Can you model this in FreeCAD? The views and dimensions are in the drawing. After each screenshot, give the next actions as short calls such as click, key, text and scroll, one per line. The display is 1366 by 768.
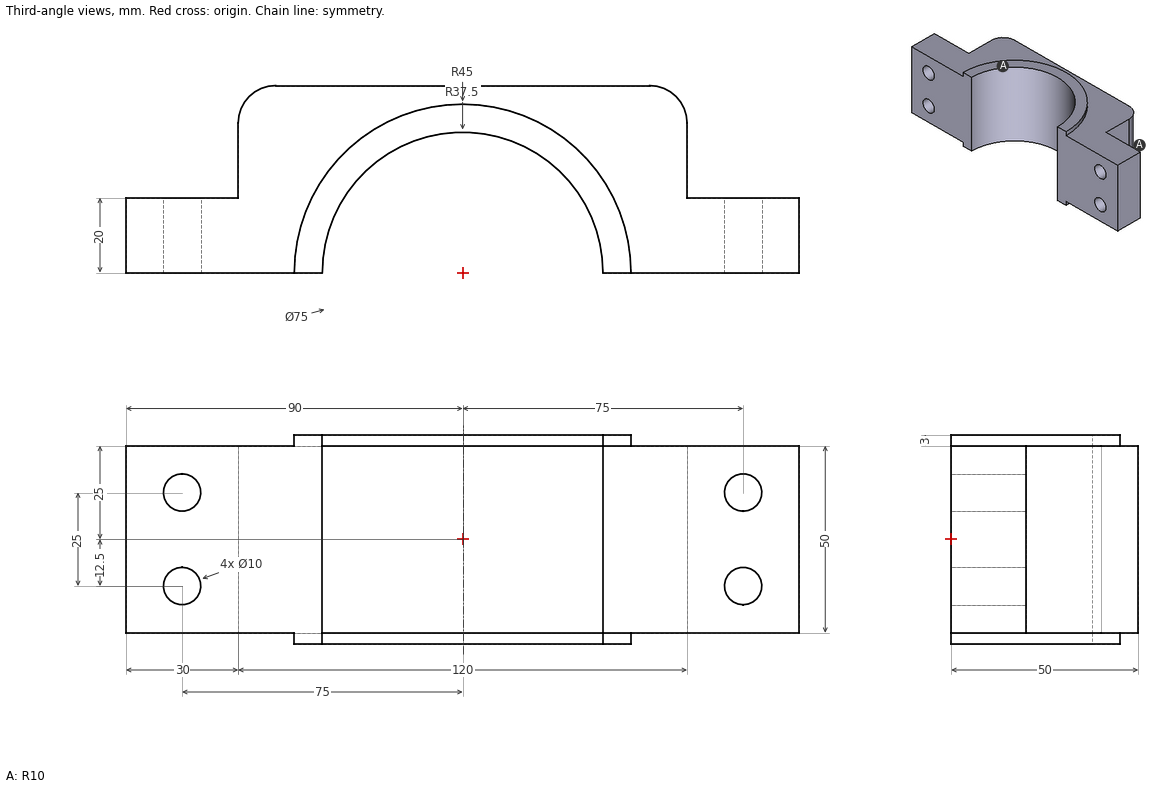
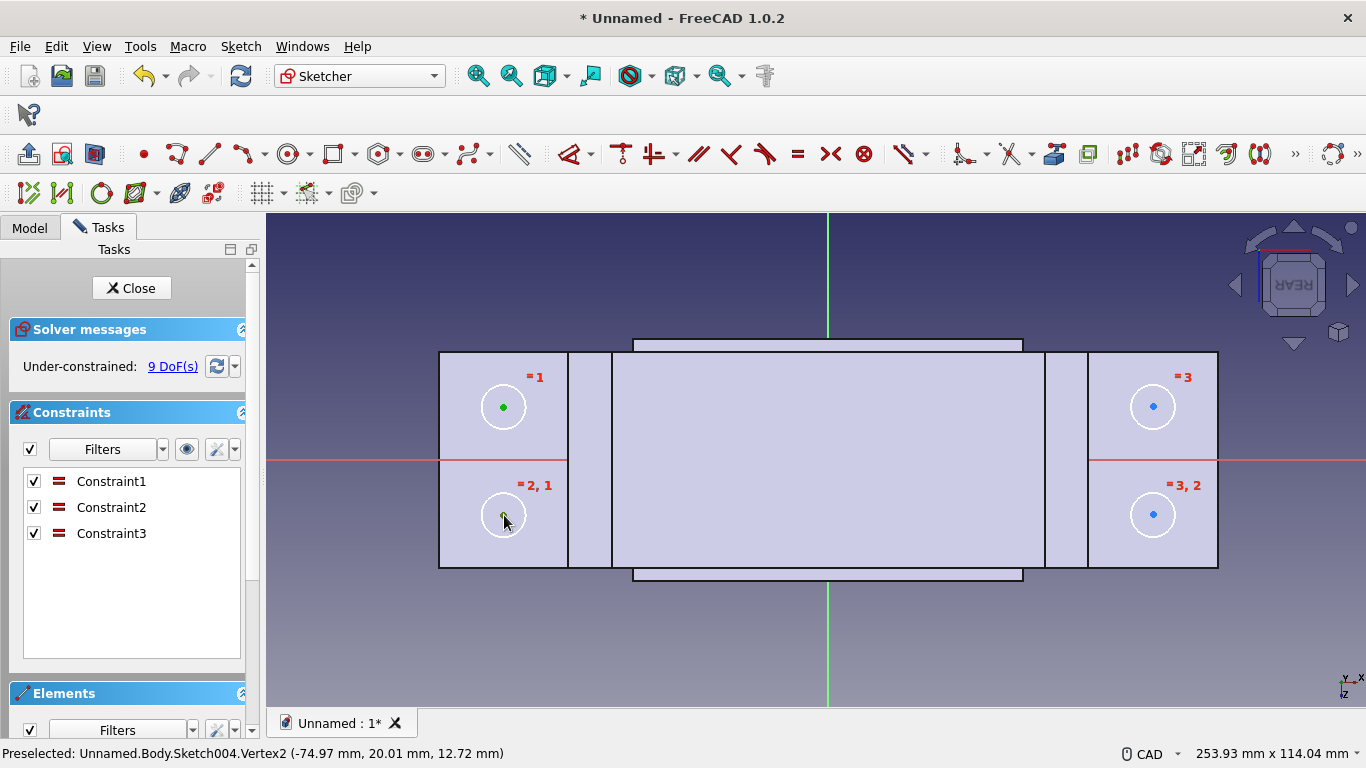
click(676, 154)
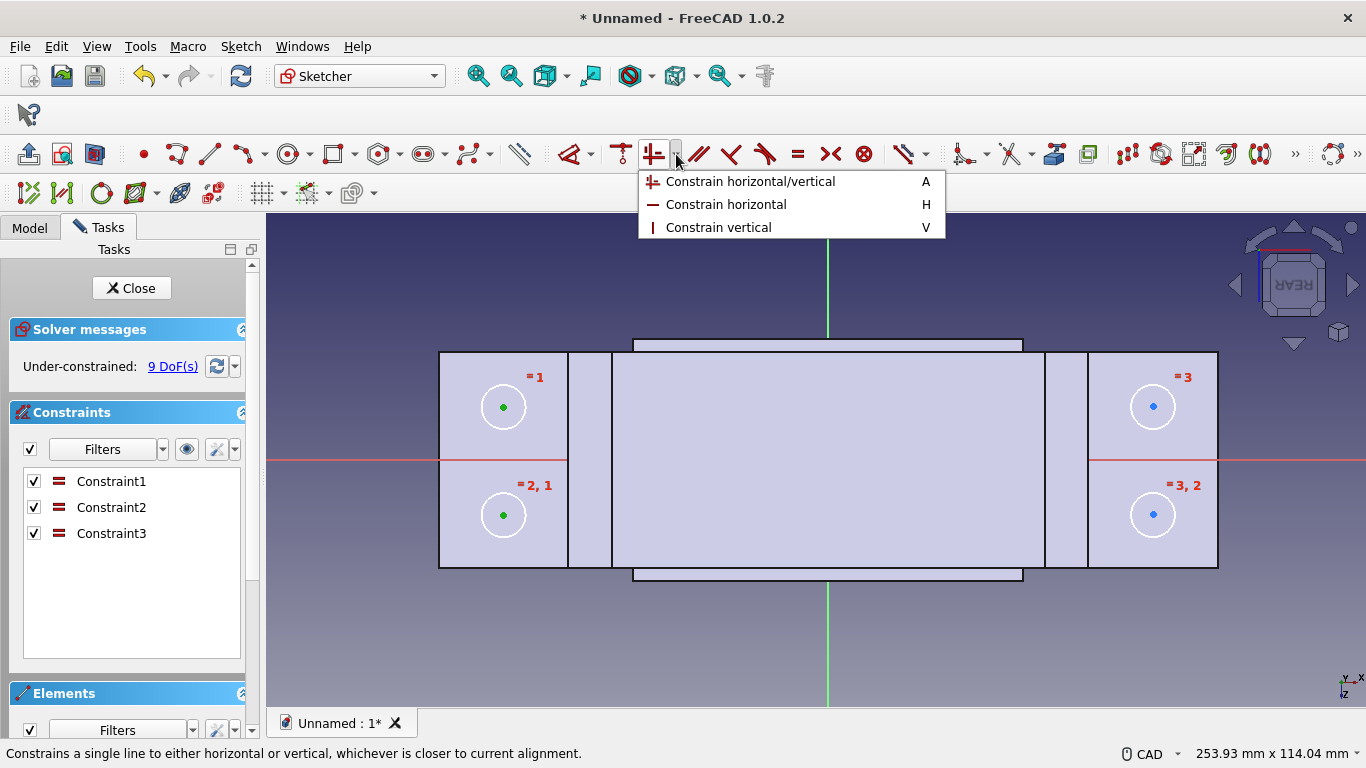
click(792, 228)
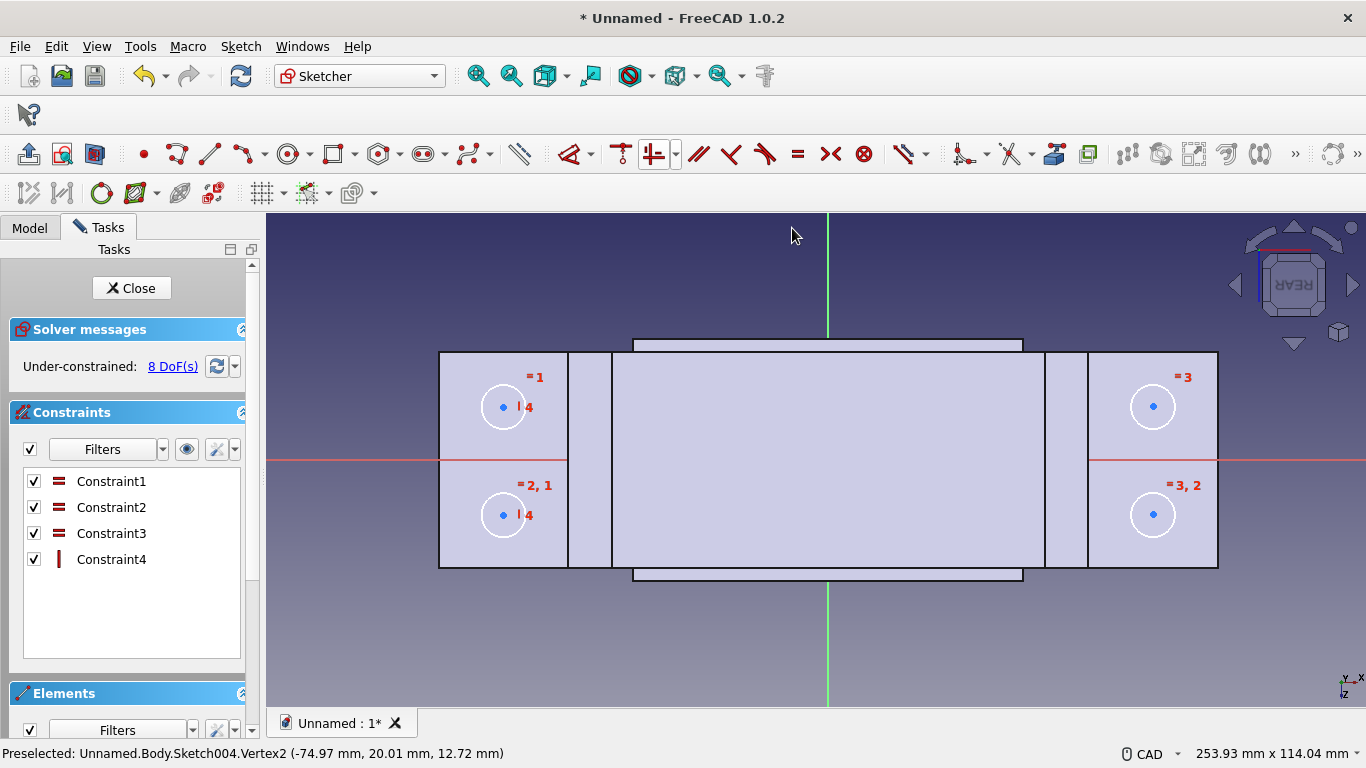
click(504, 515)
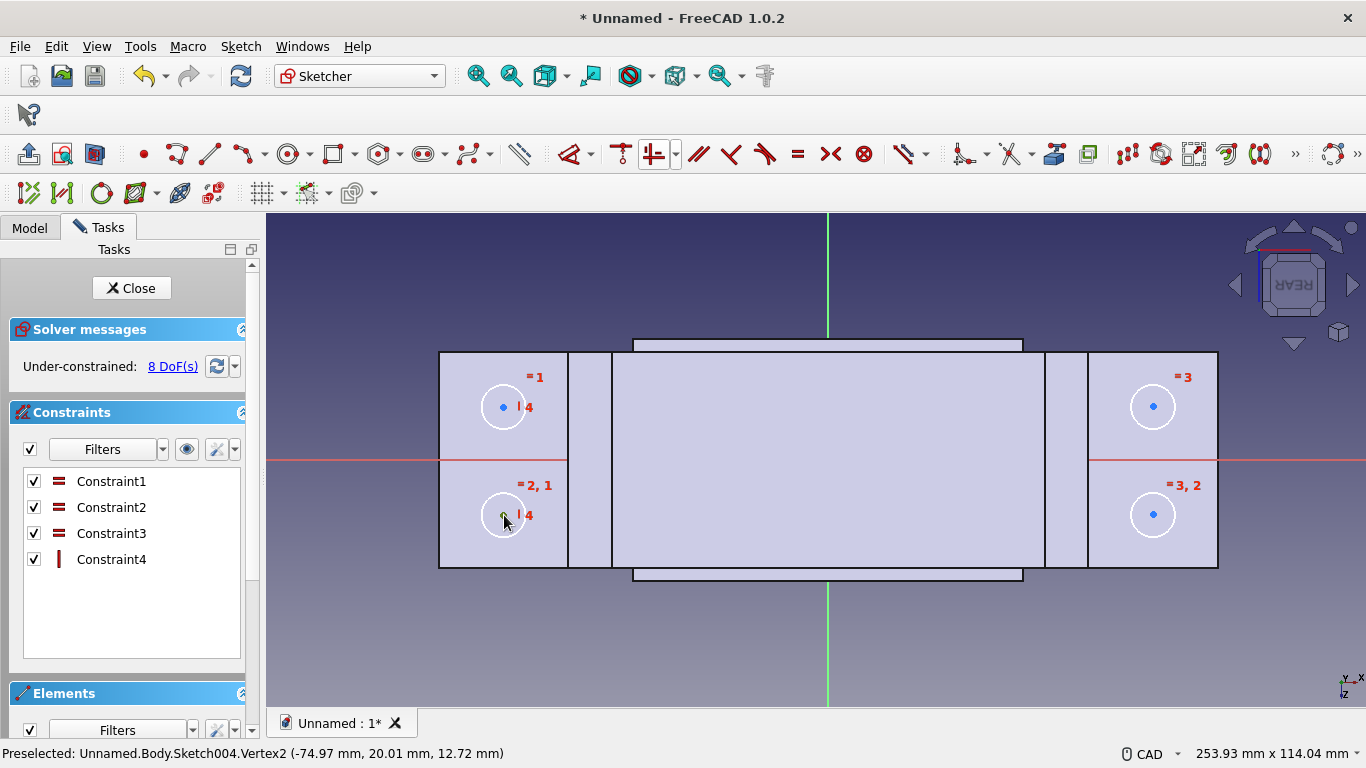
click(1153, 515)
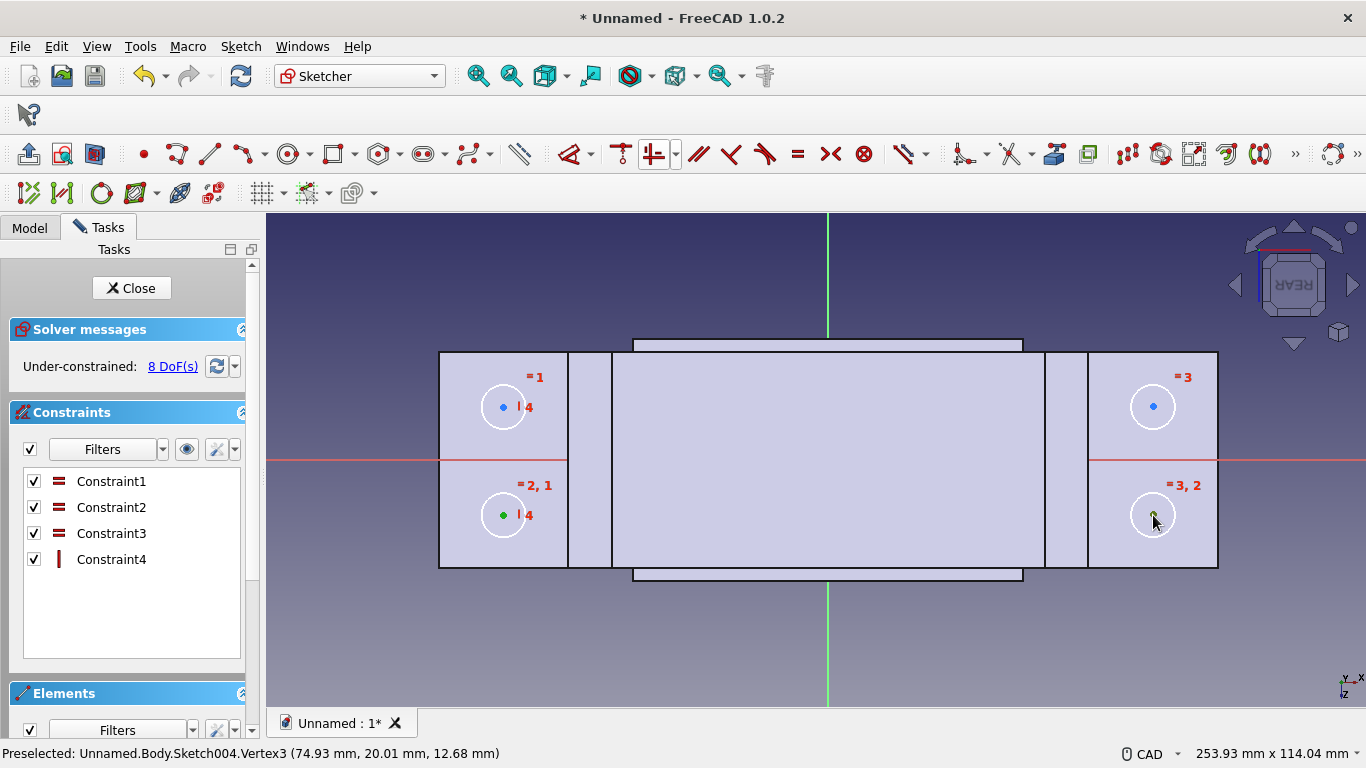
click(676, 154)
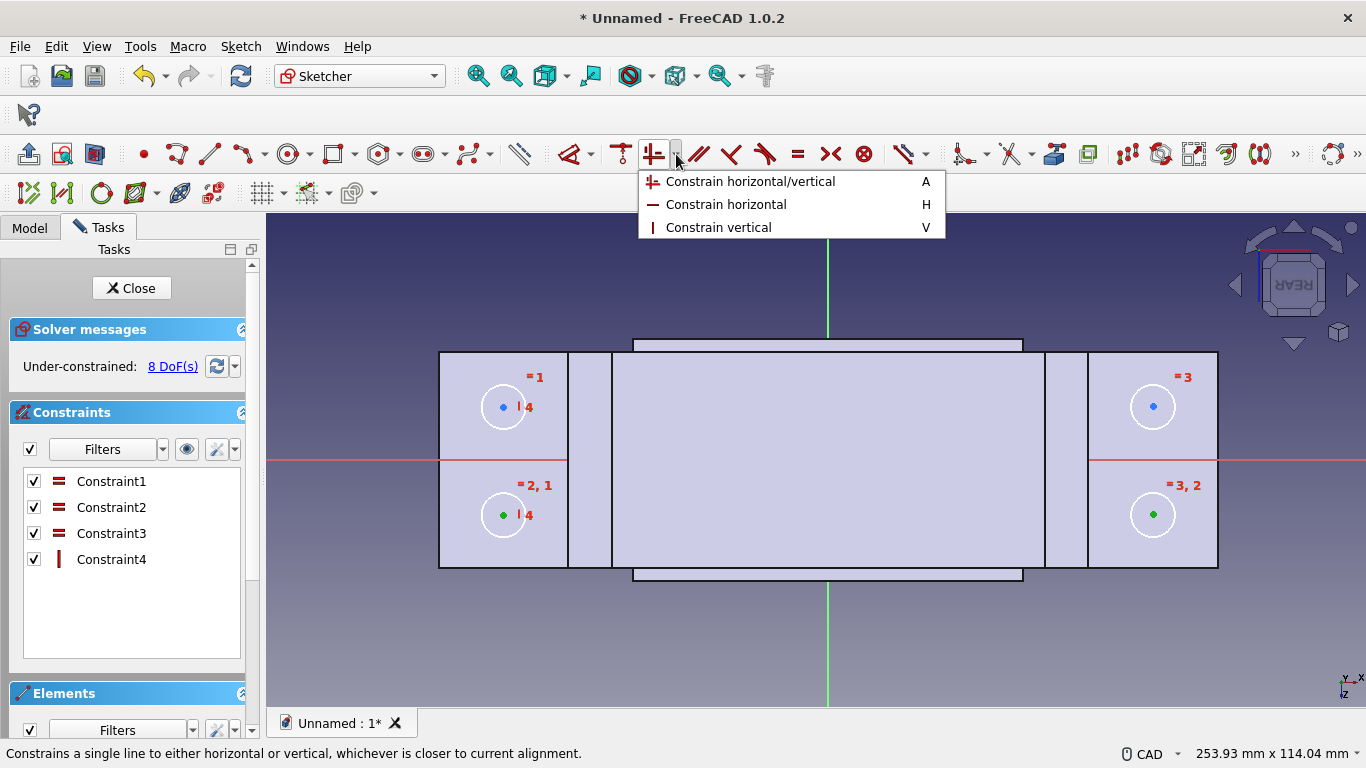
click(792, 204)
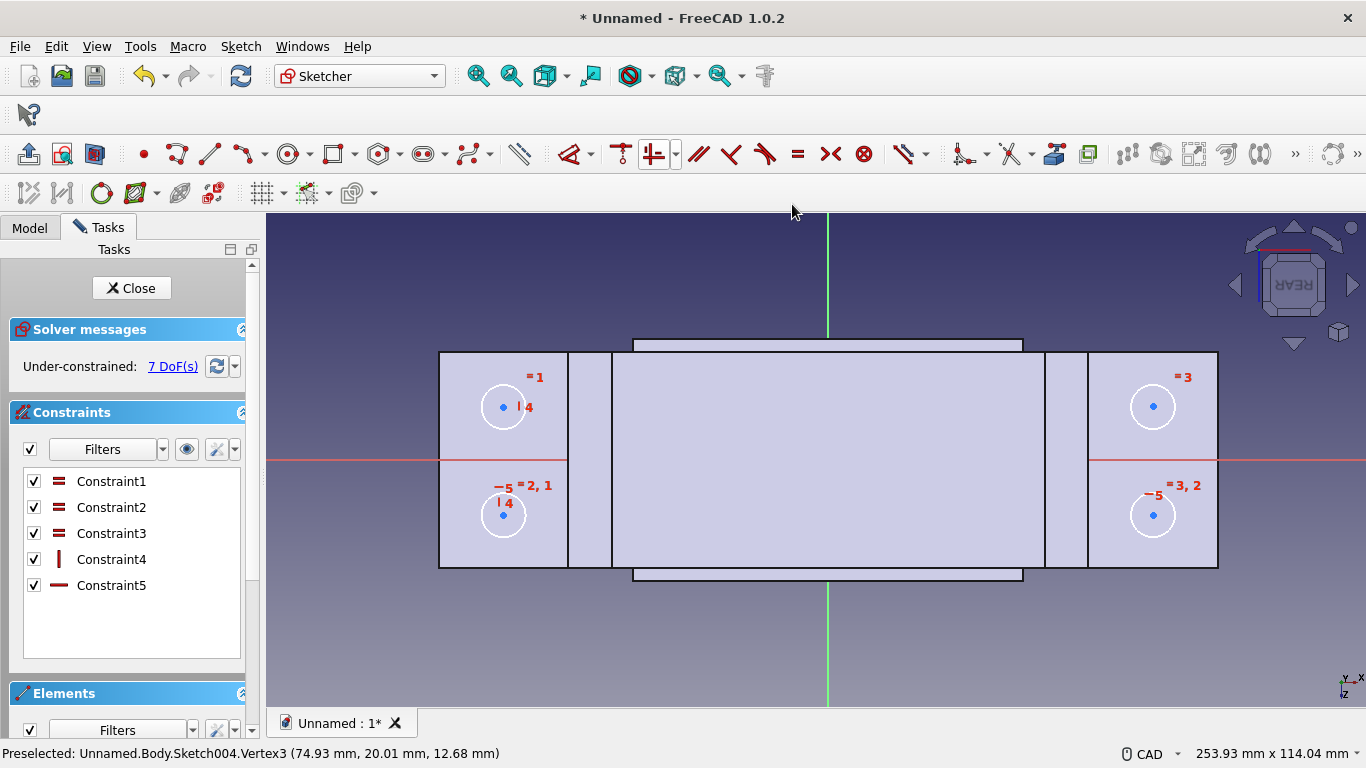
click(1153, 515)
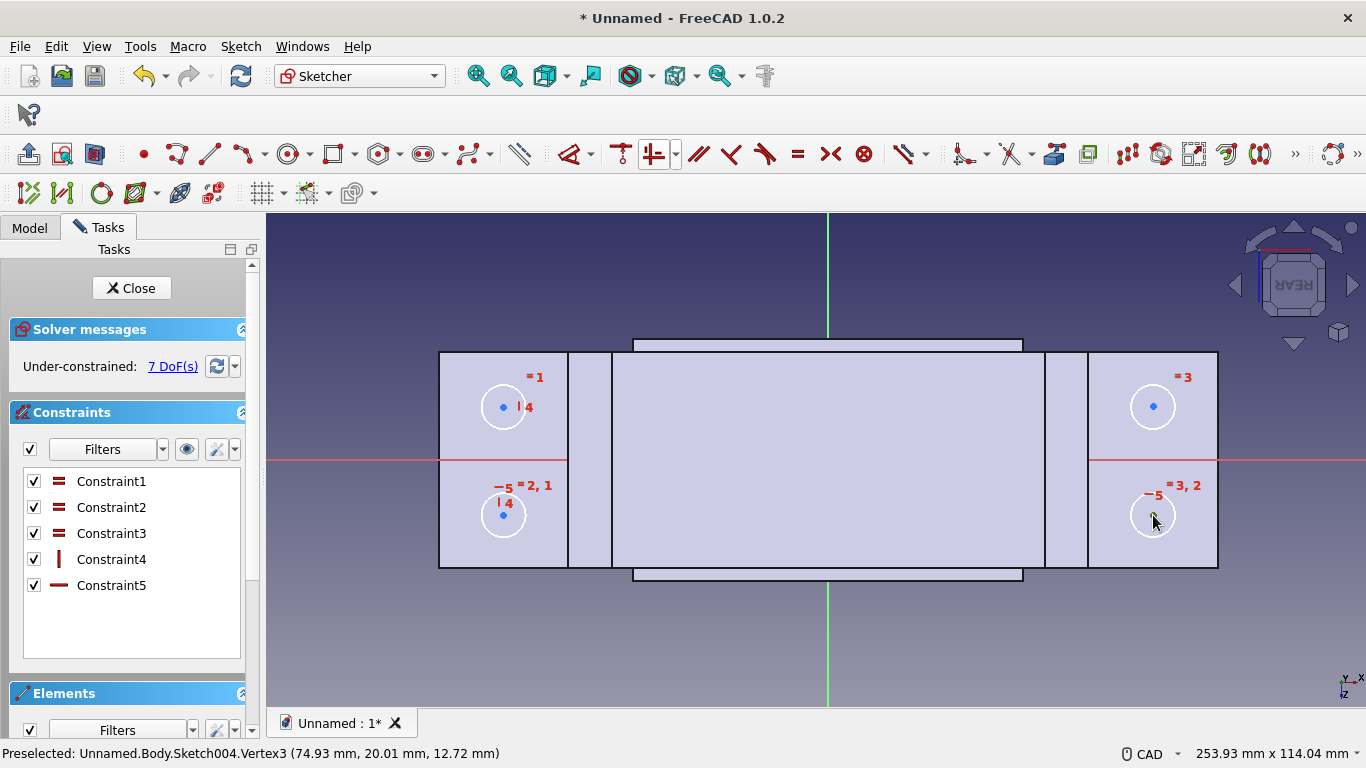
click(1153, 407)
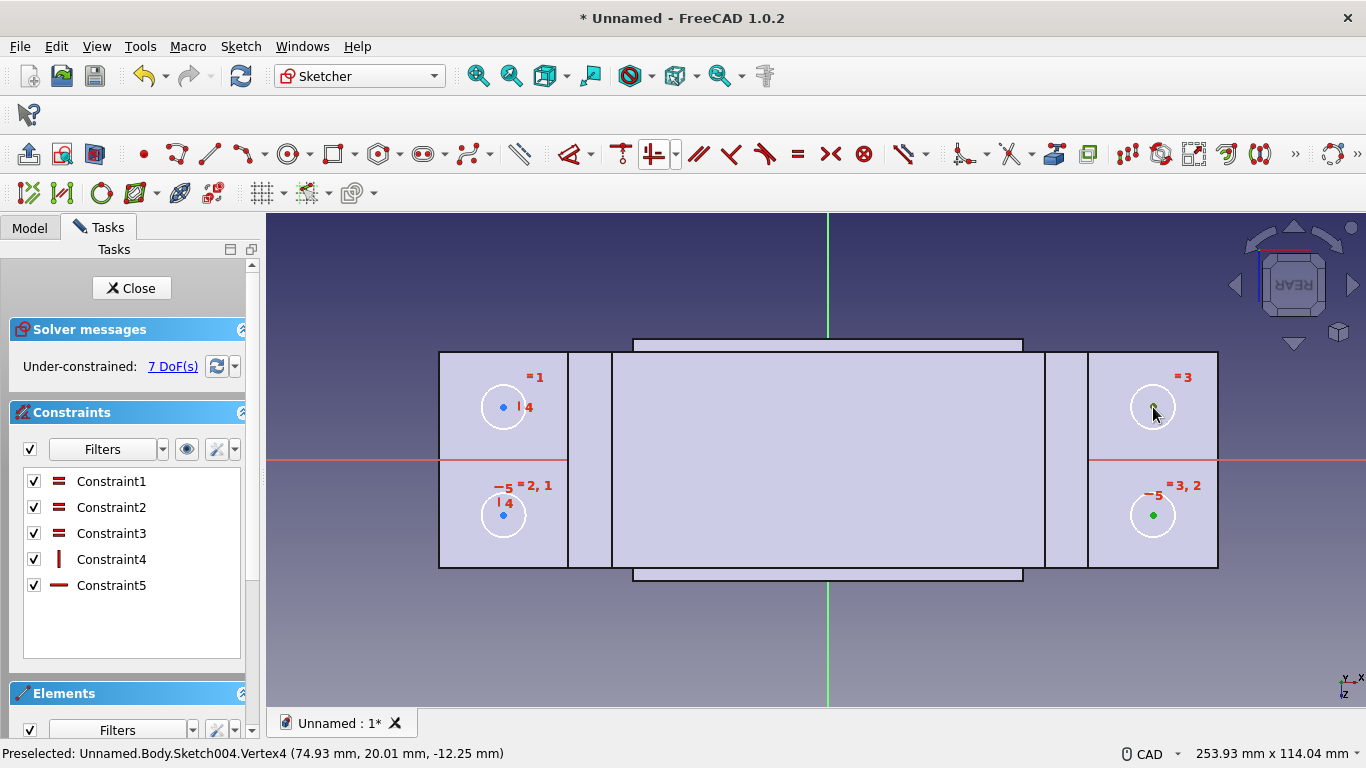
key(v)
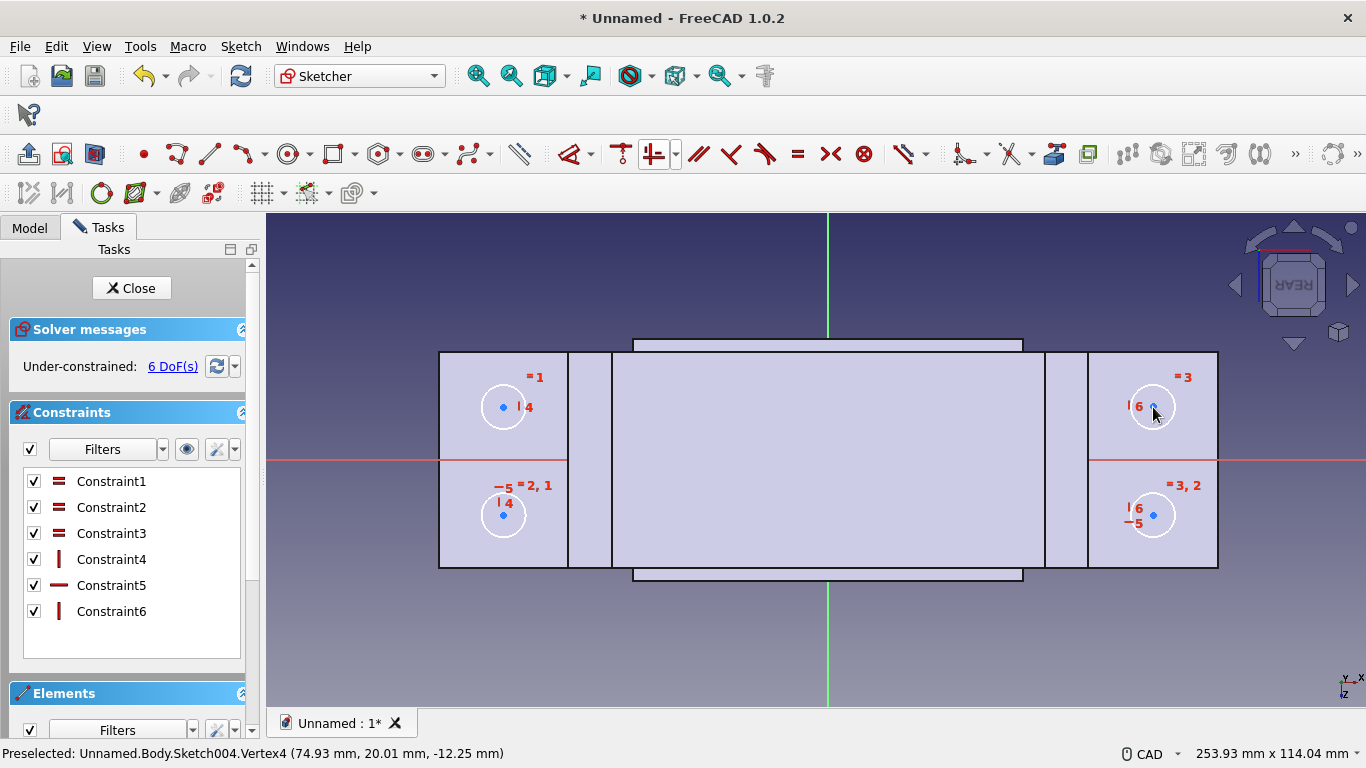
click(504, 407)